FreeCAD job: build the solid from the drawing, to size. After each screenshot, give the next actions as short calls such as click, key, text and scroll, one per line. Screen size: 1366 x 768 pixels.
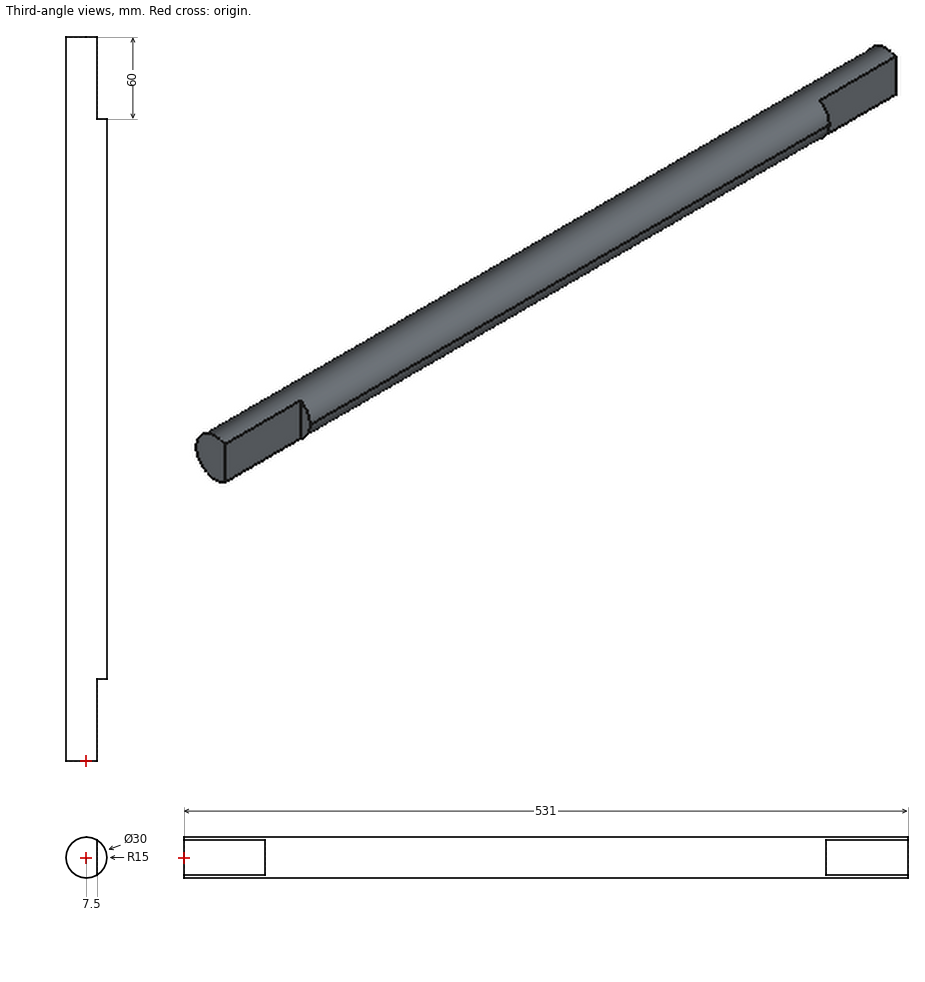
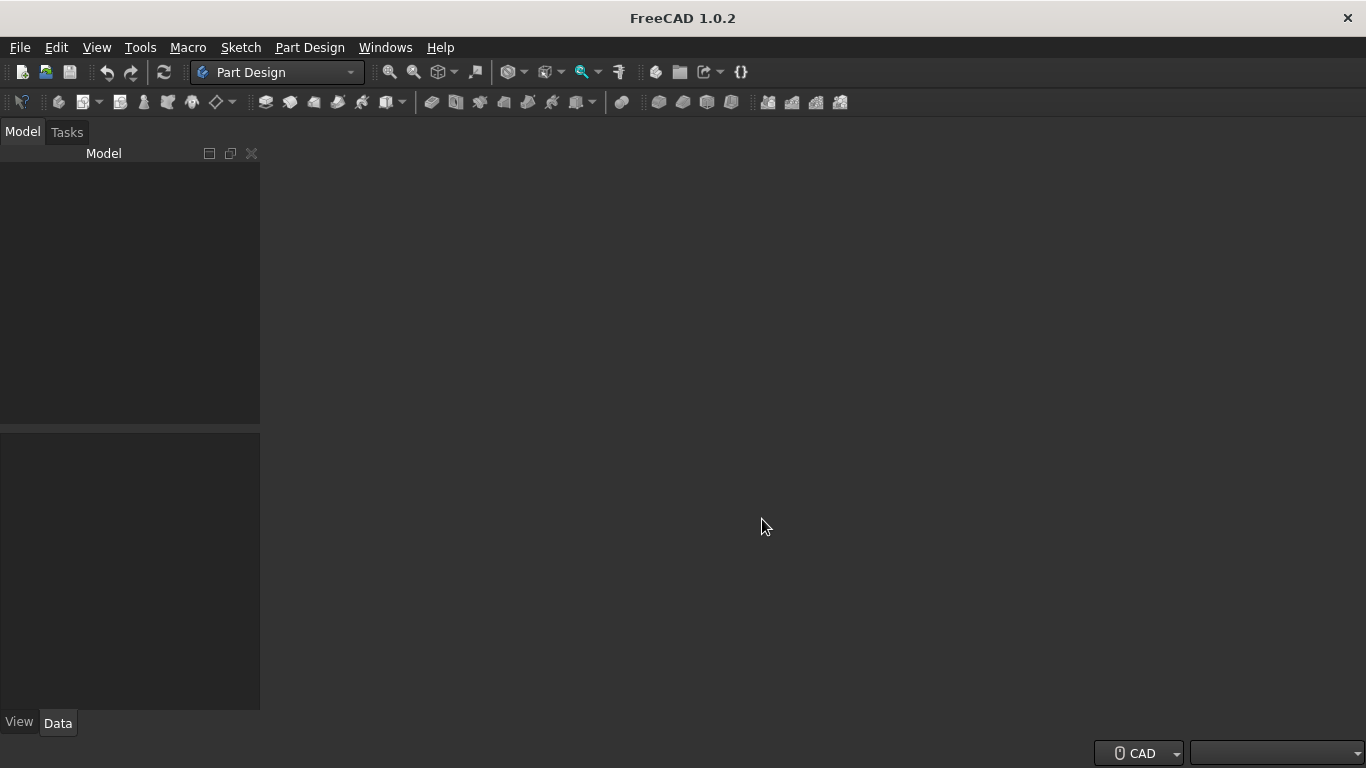
click(22, 72)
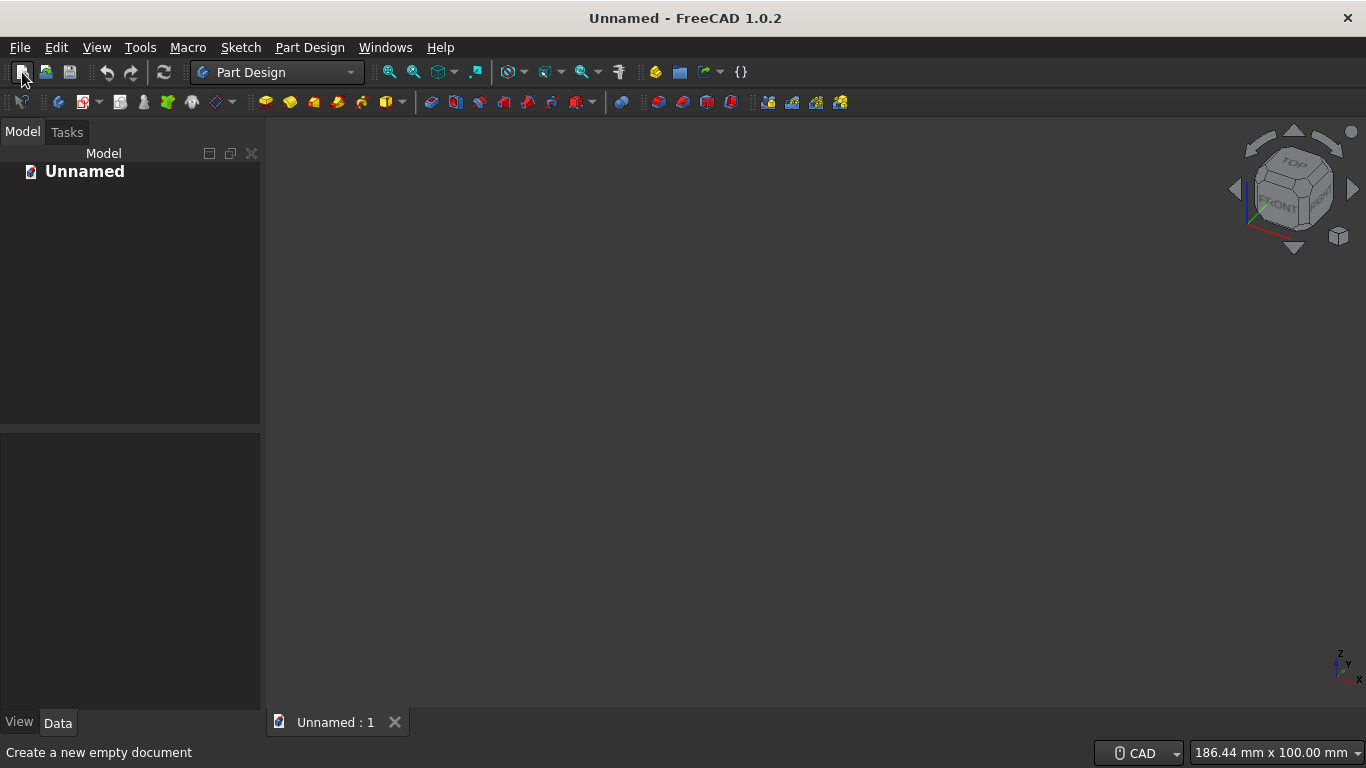
click(84, 102)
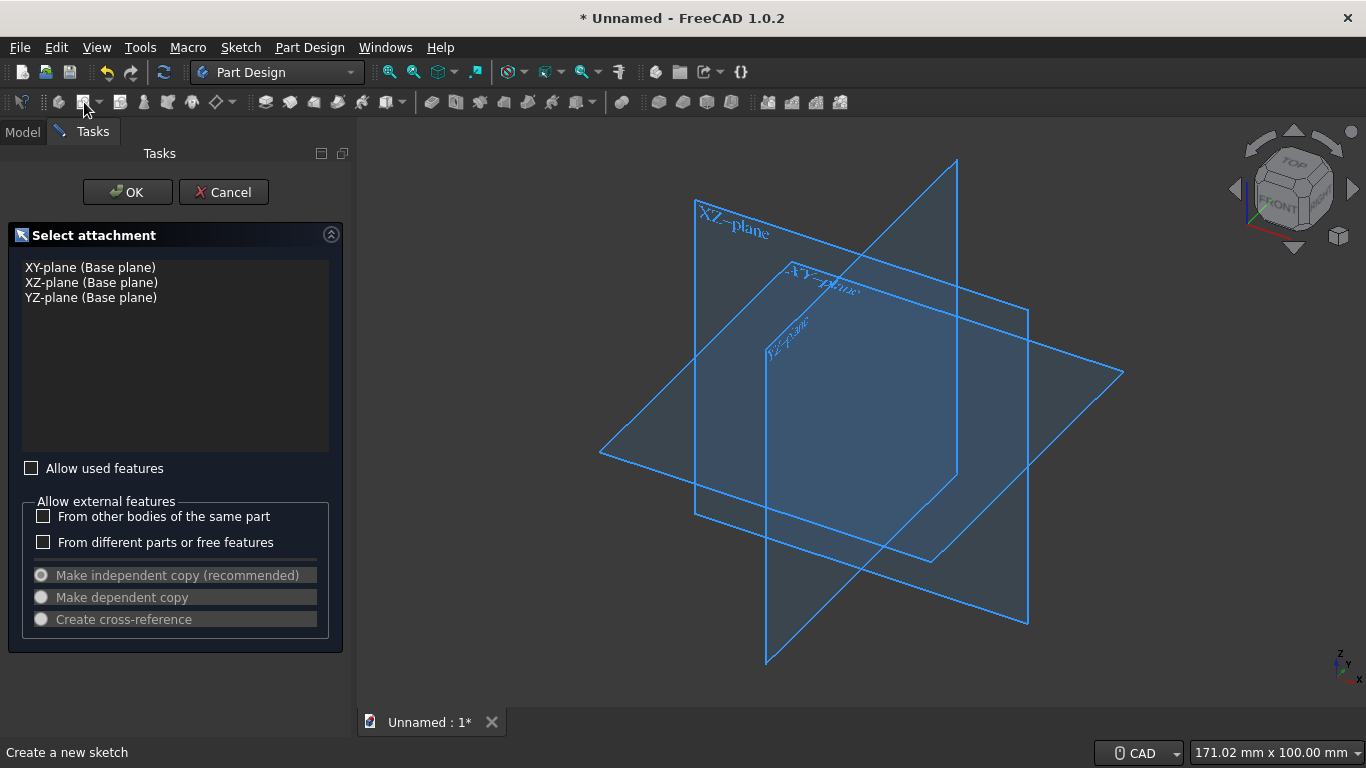
click(82, 282)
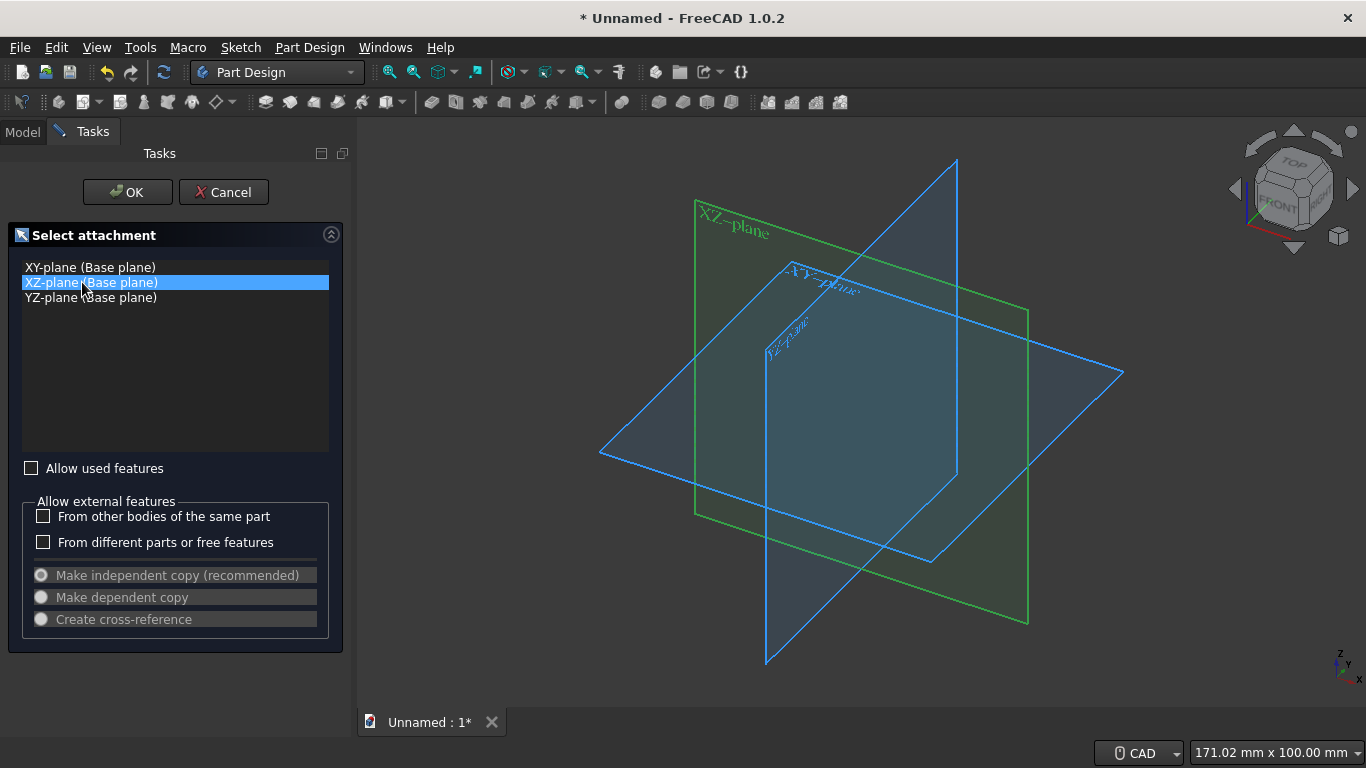
click(128, 192)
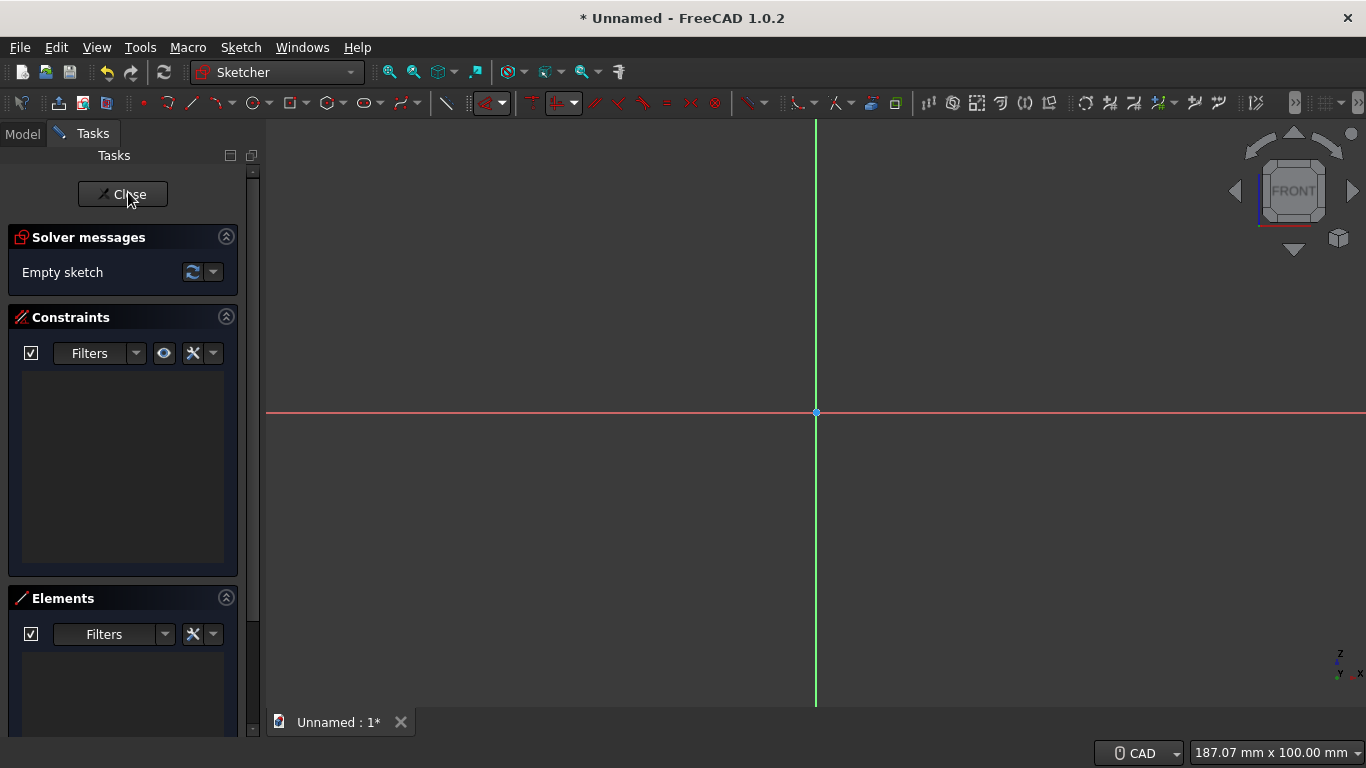
scroll(872, 413, up, 4)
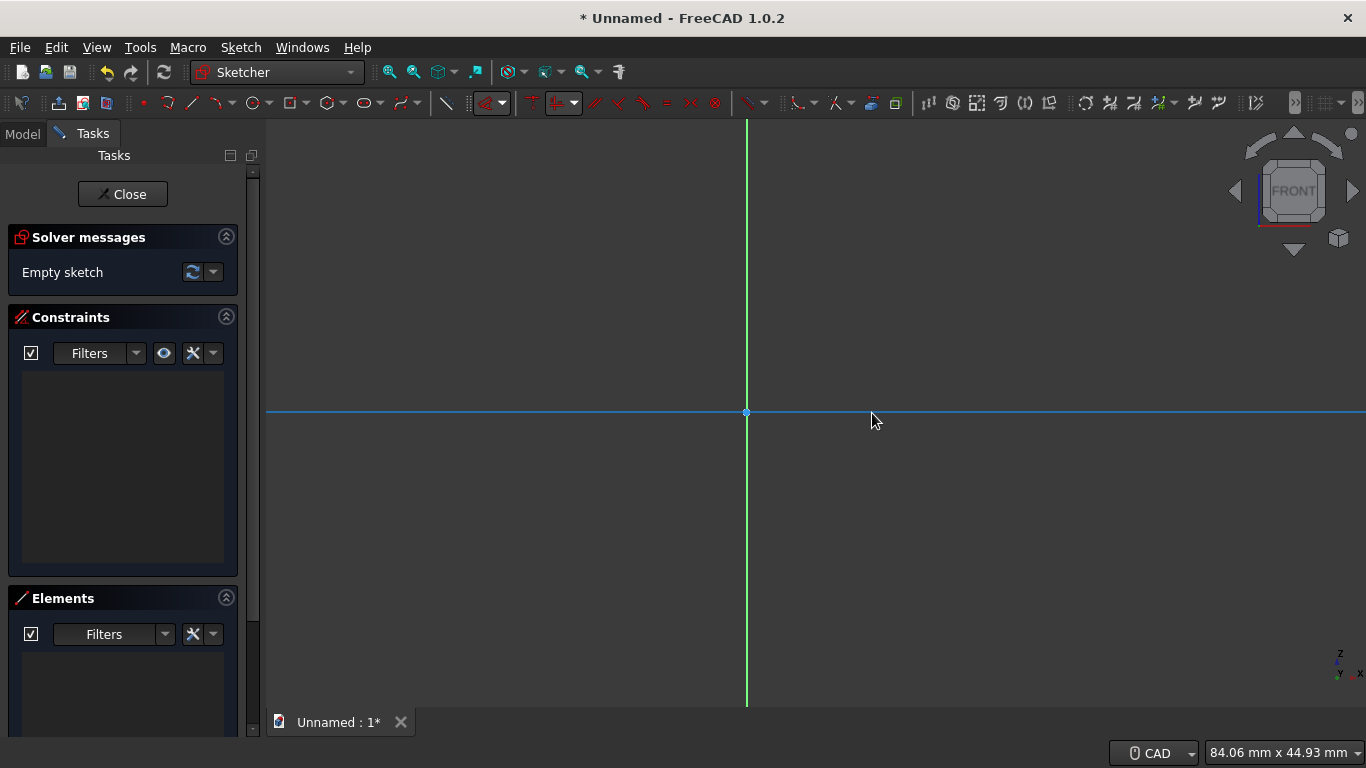
click(254, 104)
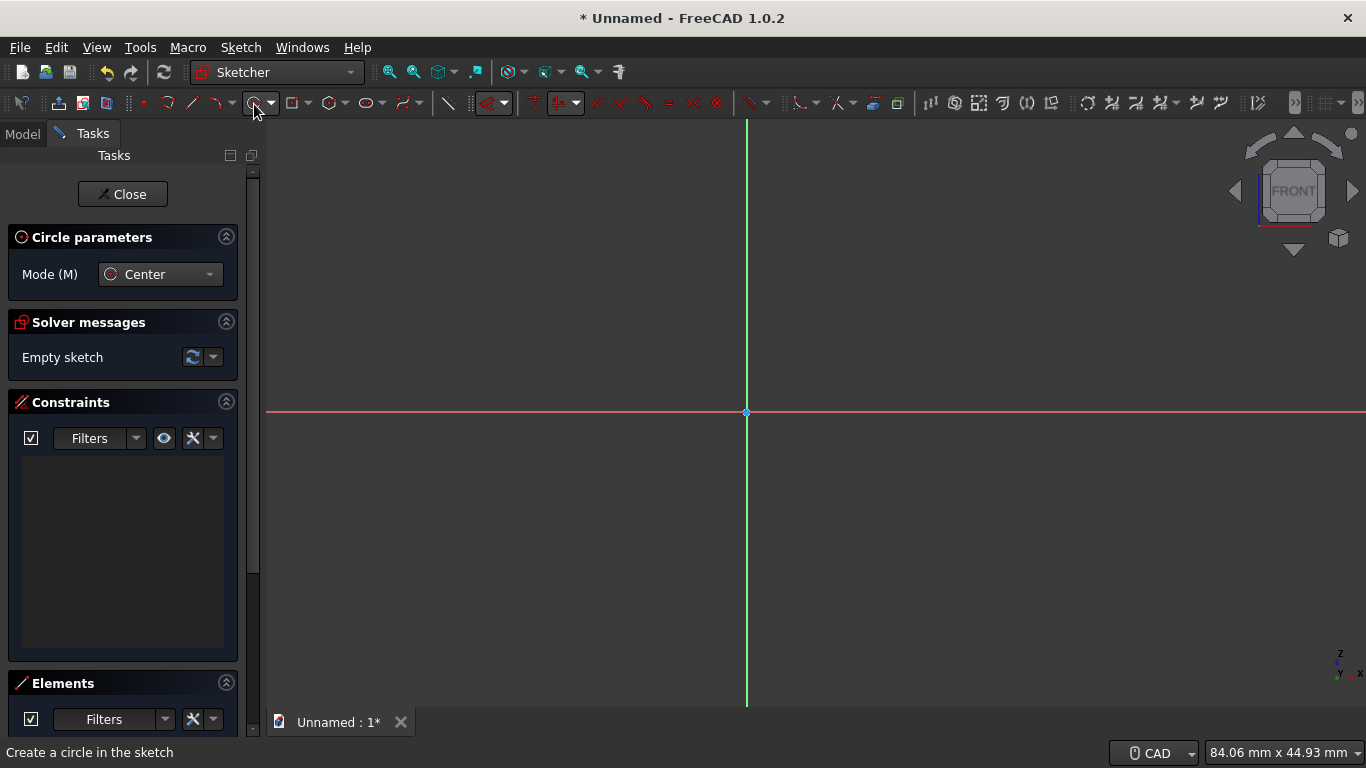
click(747, 412)
move(885, 274)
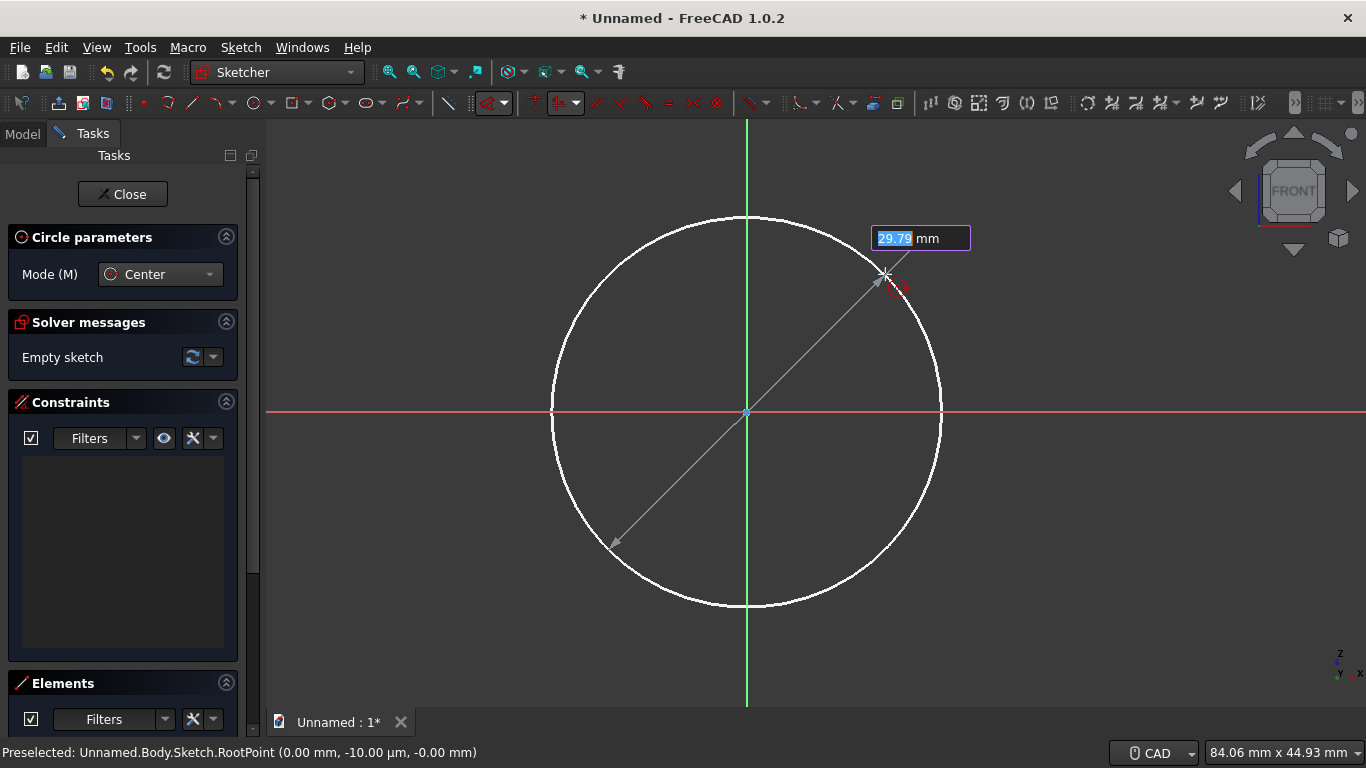
text(30)
key(Return)
key(Escape)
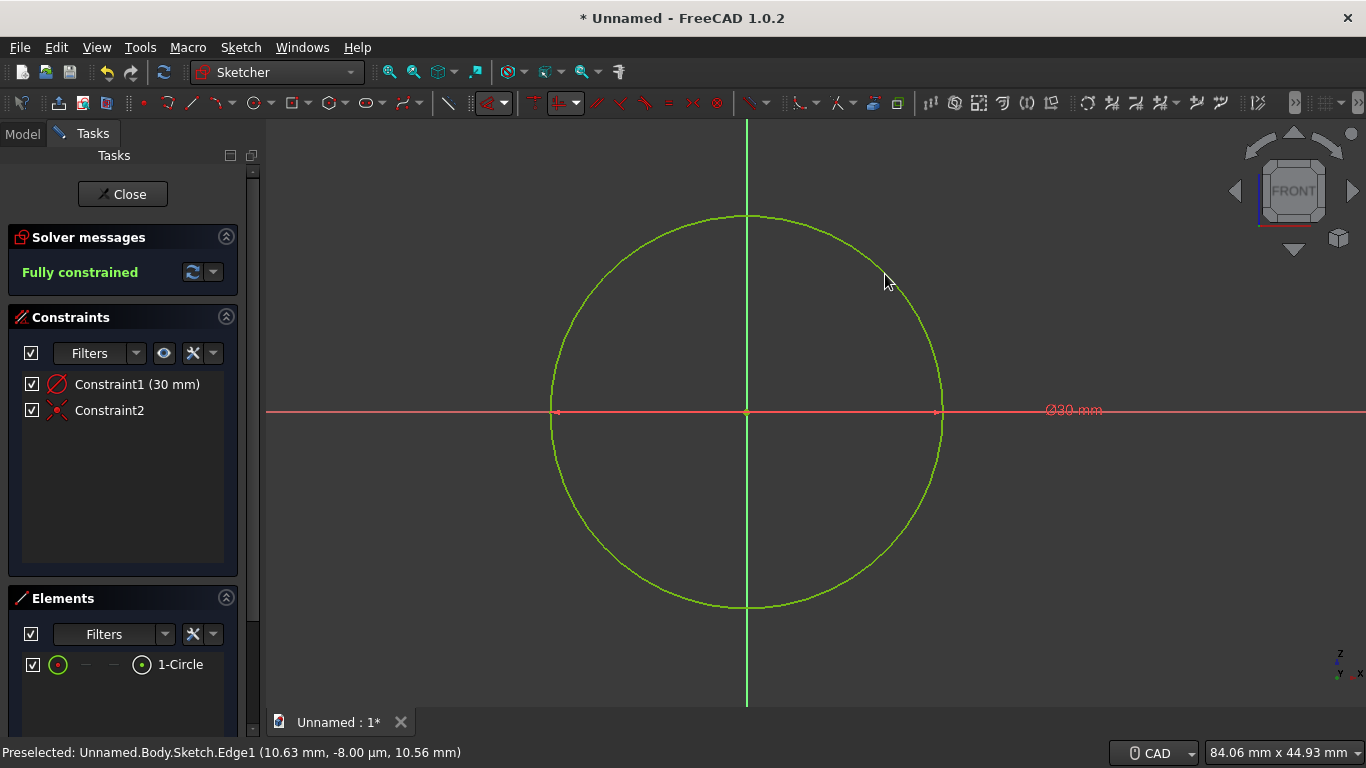
click(123, 194)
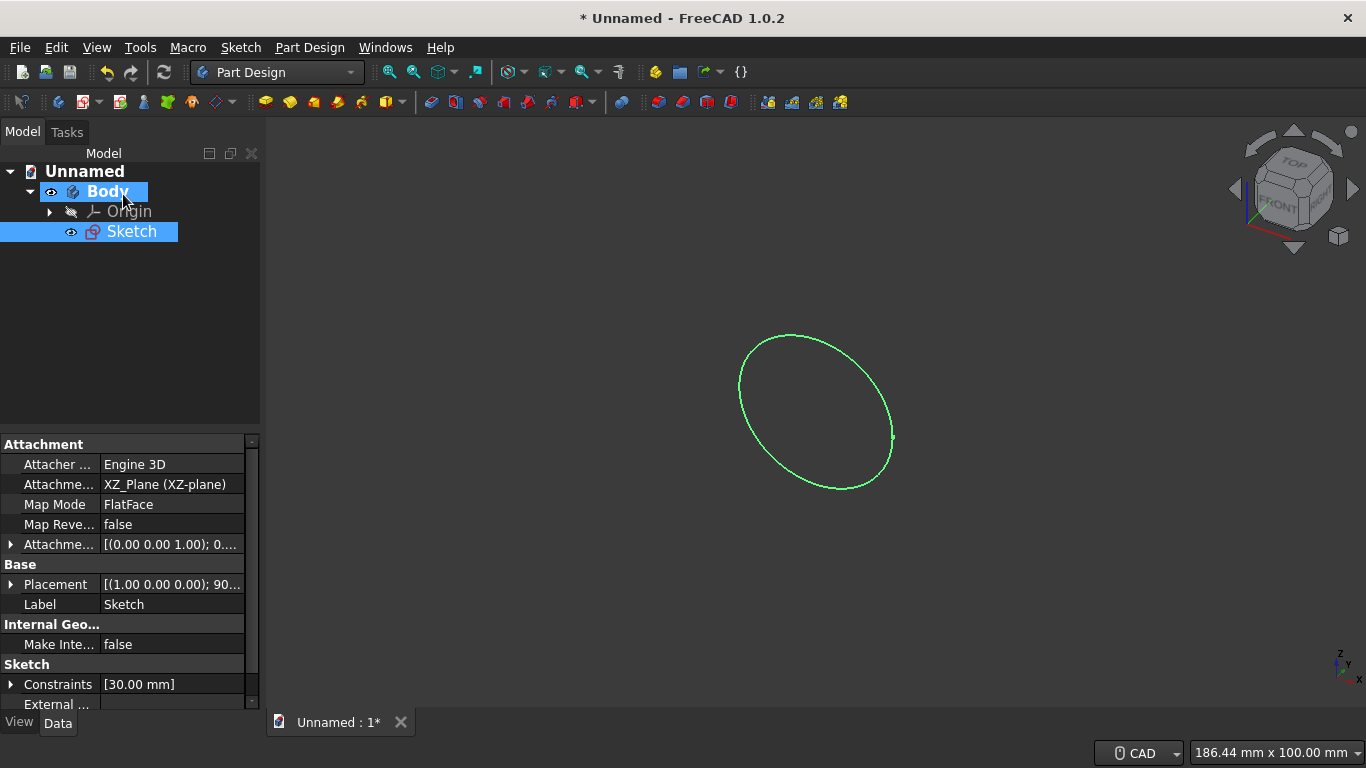
click(266, 102)